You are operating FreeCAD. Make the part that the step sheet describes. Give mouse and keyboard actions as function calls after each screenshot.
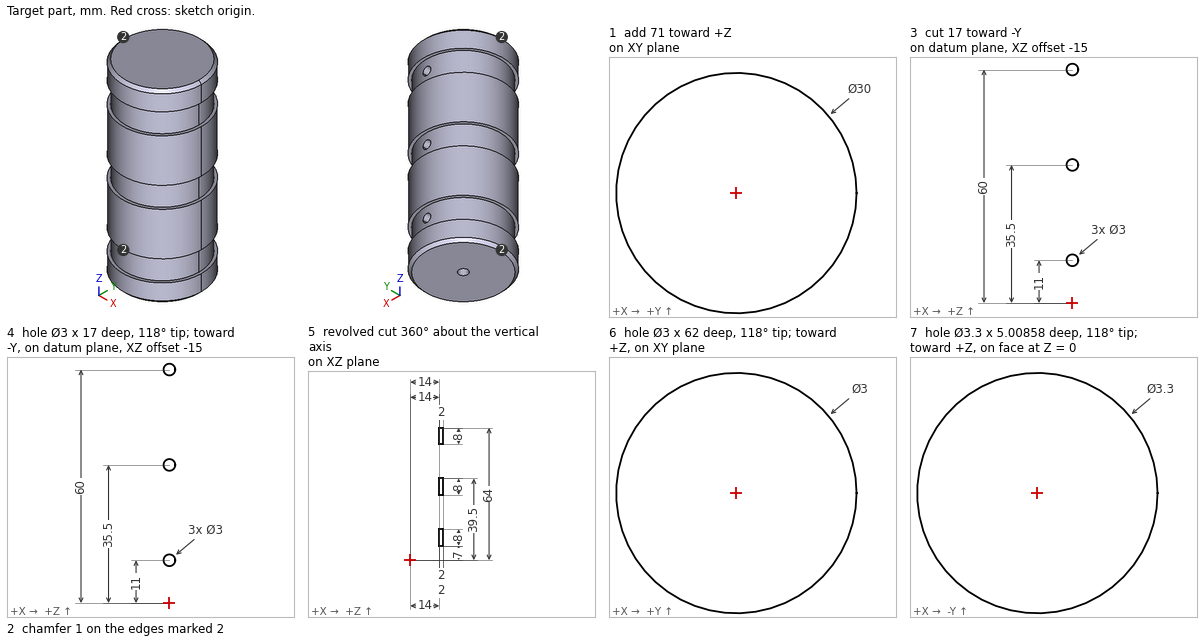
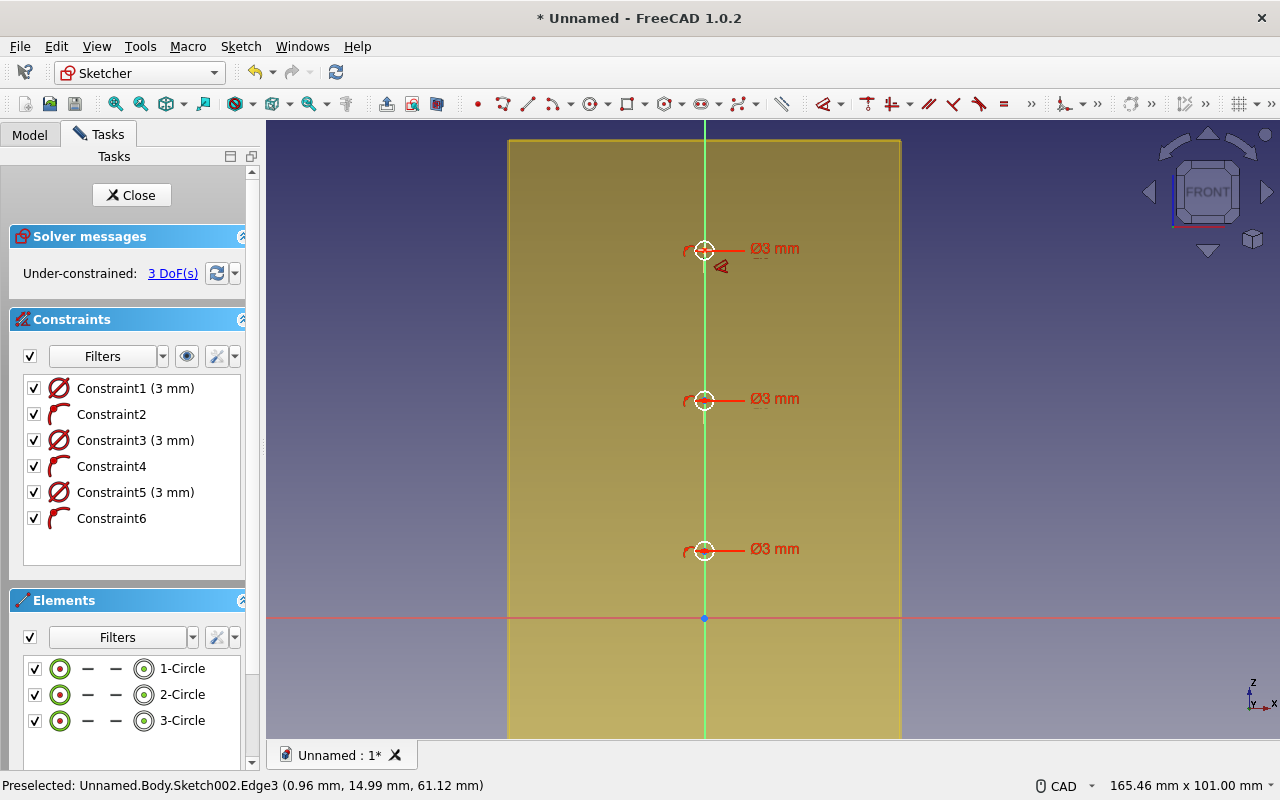
click(705, 551)
click(739, 585)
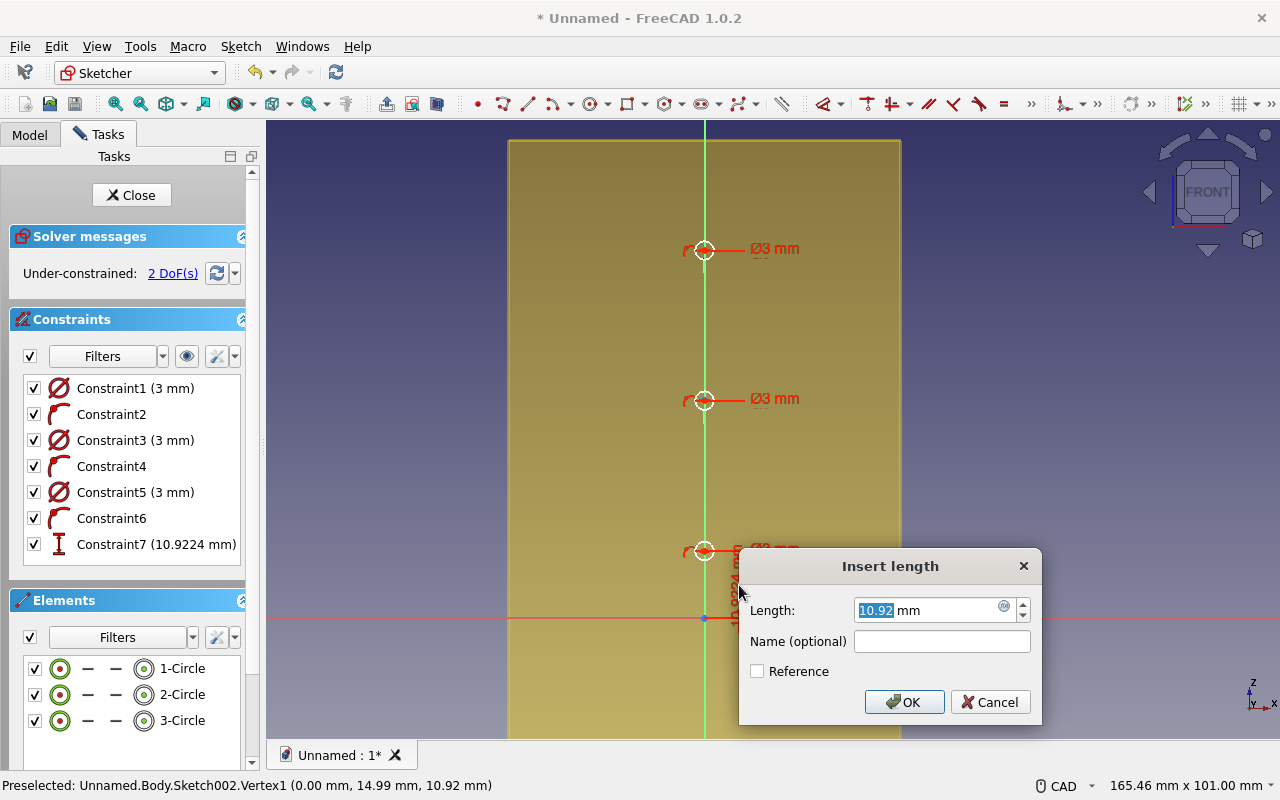
text(11)
key(Return)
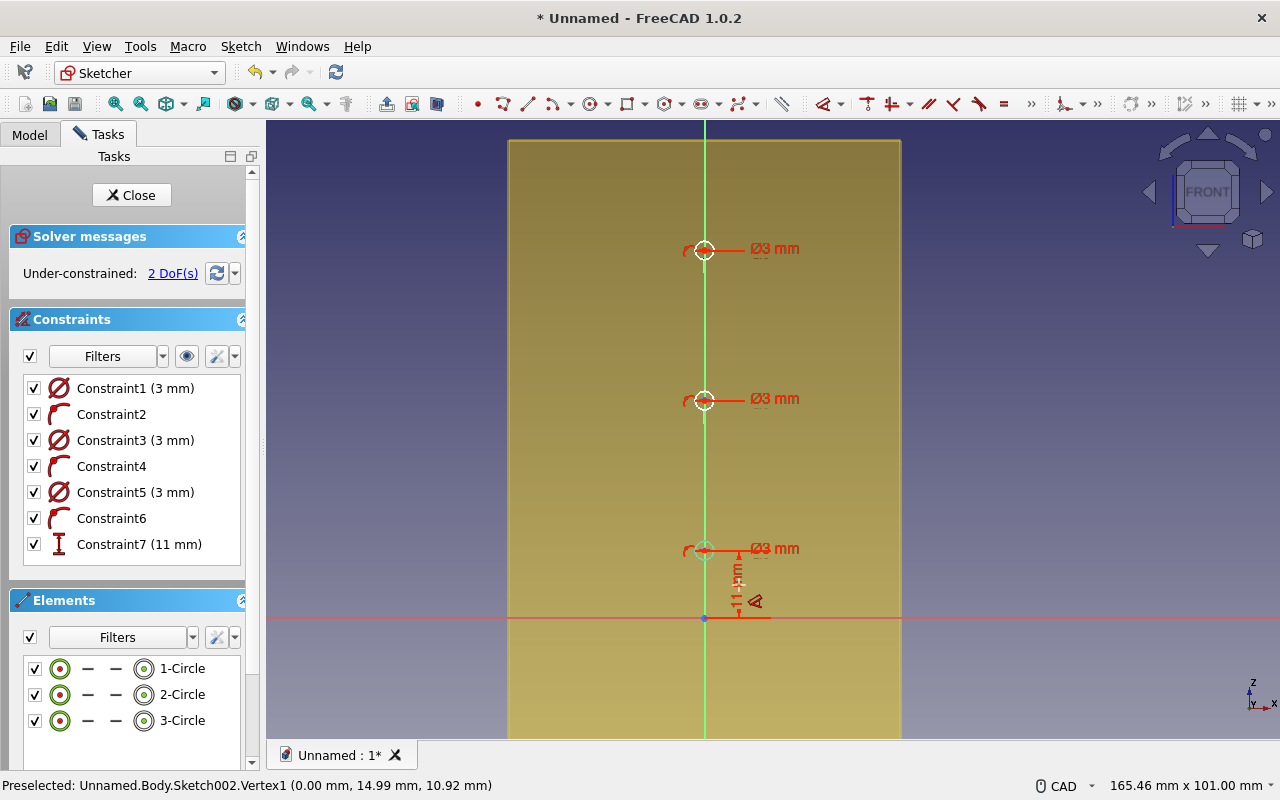
click(705, 251)
click(739, 434)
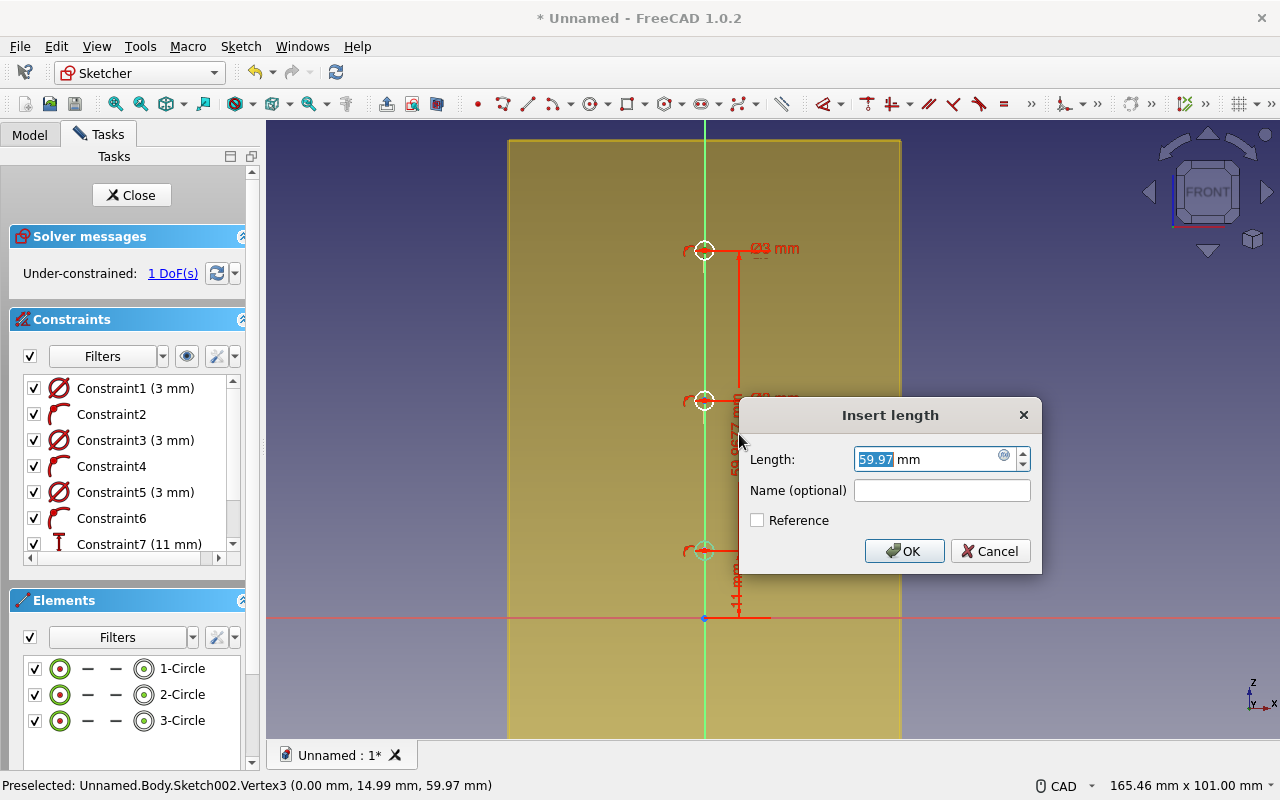
text(60)
key(Return)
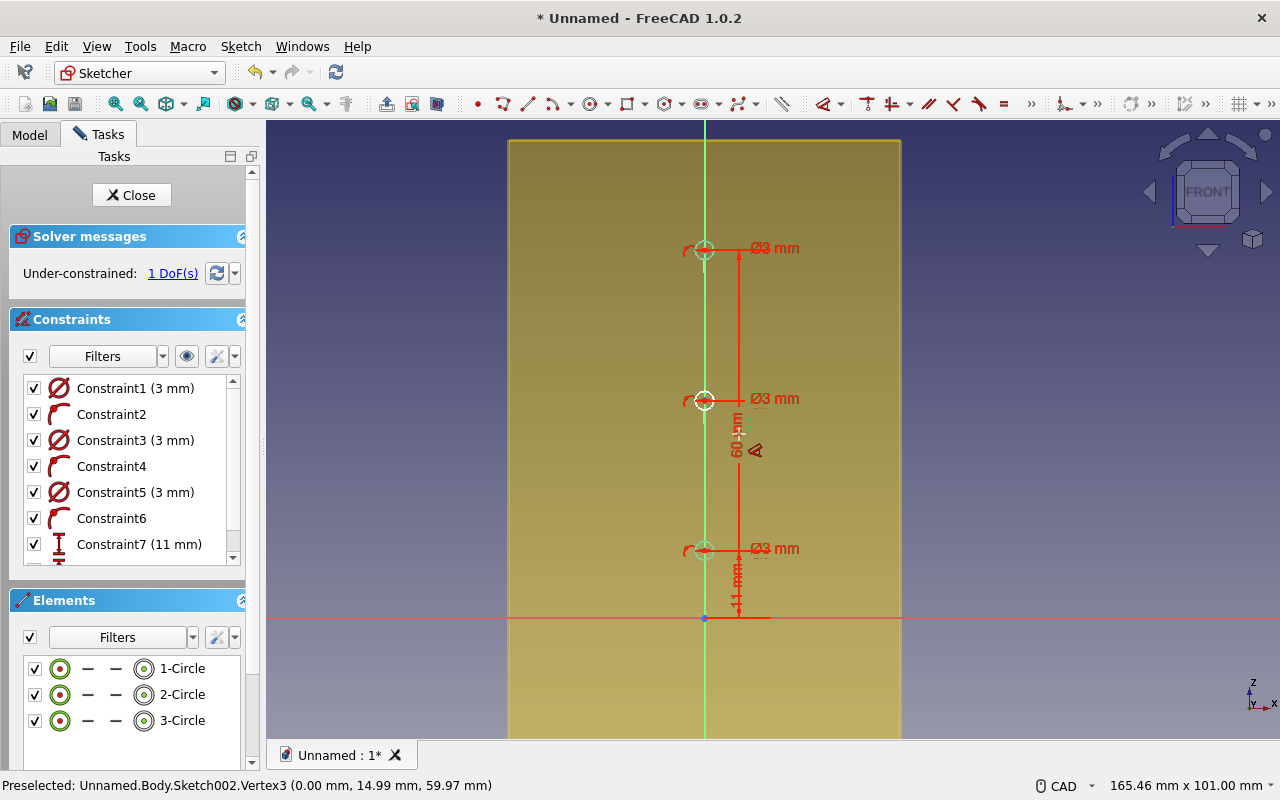
click(705, 401)
click(739, 509)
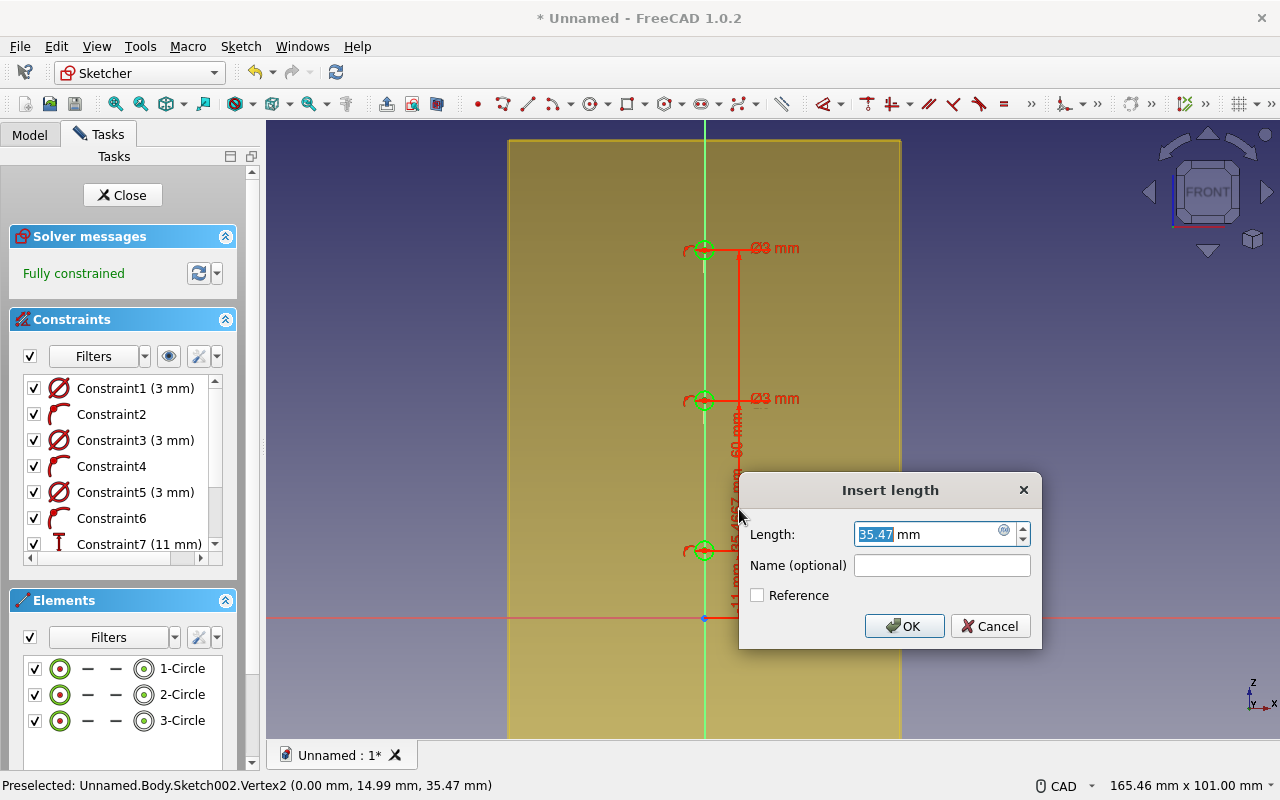
text(35.5)
key(Return)
key(Escape)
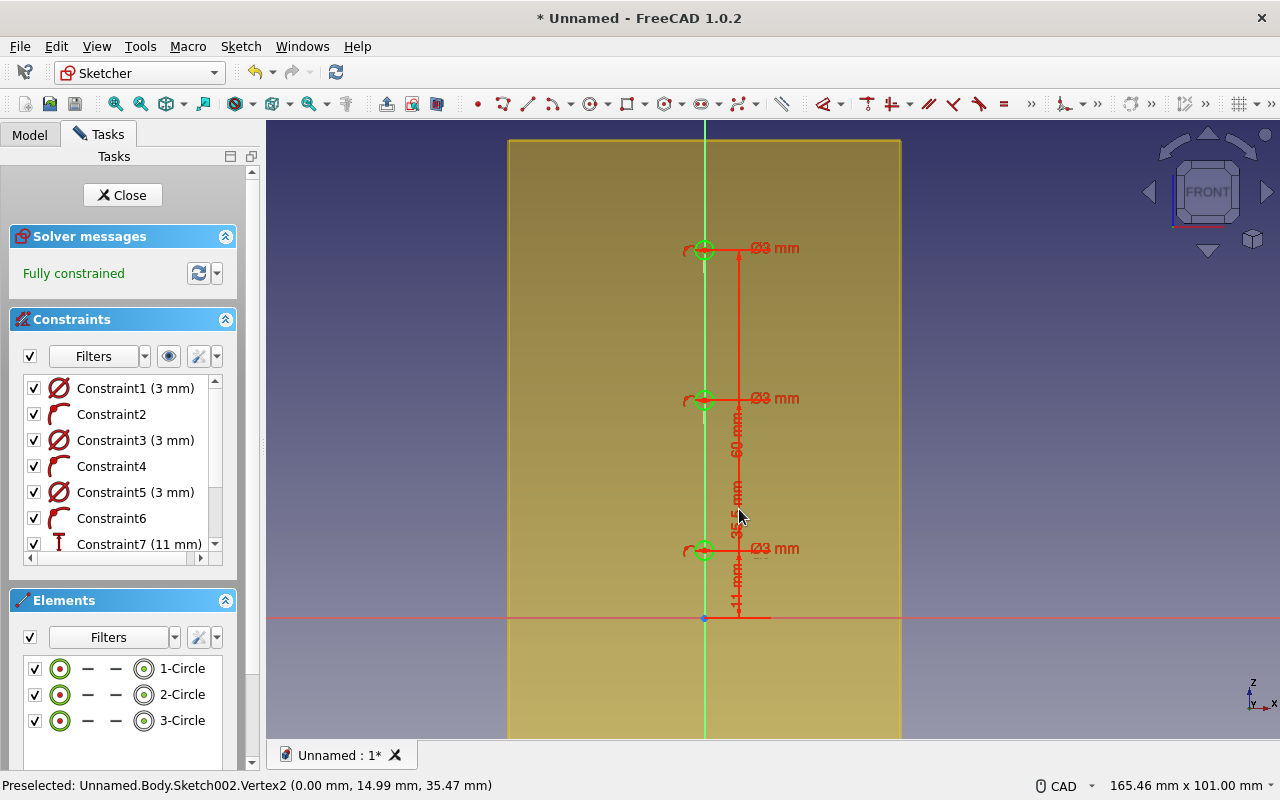
click(123, 195)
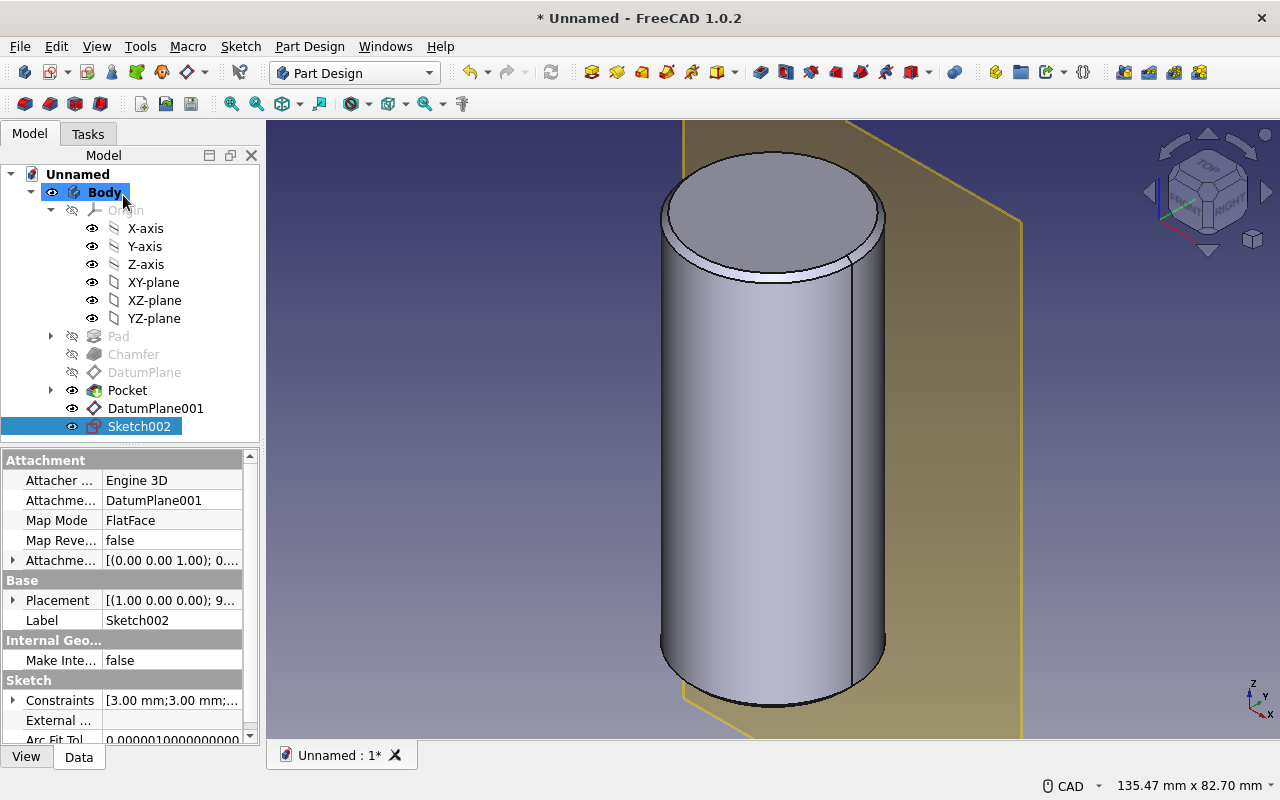
click(786, 72)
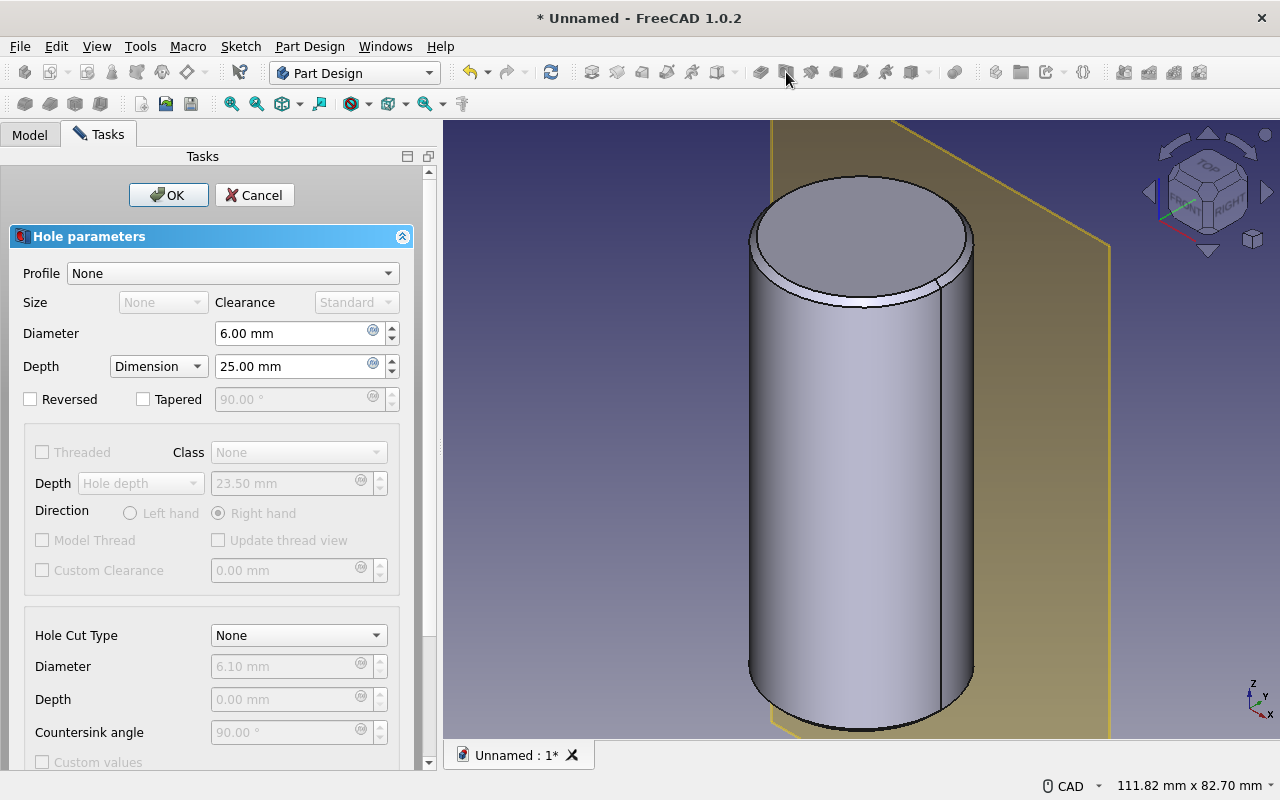
triple_click(300, 334)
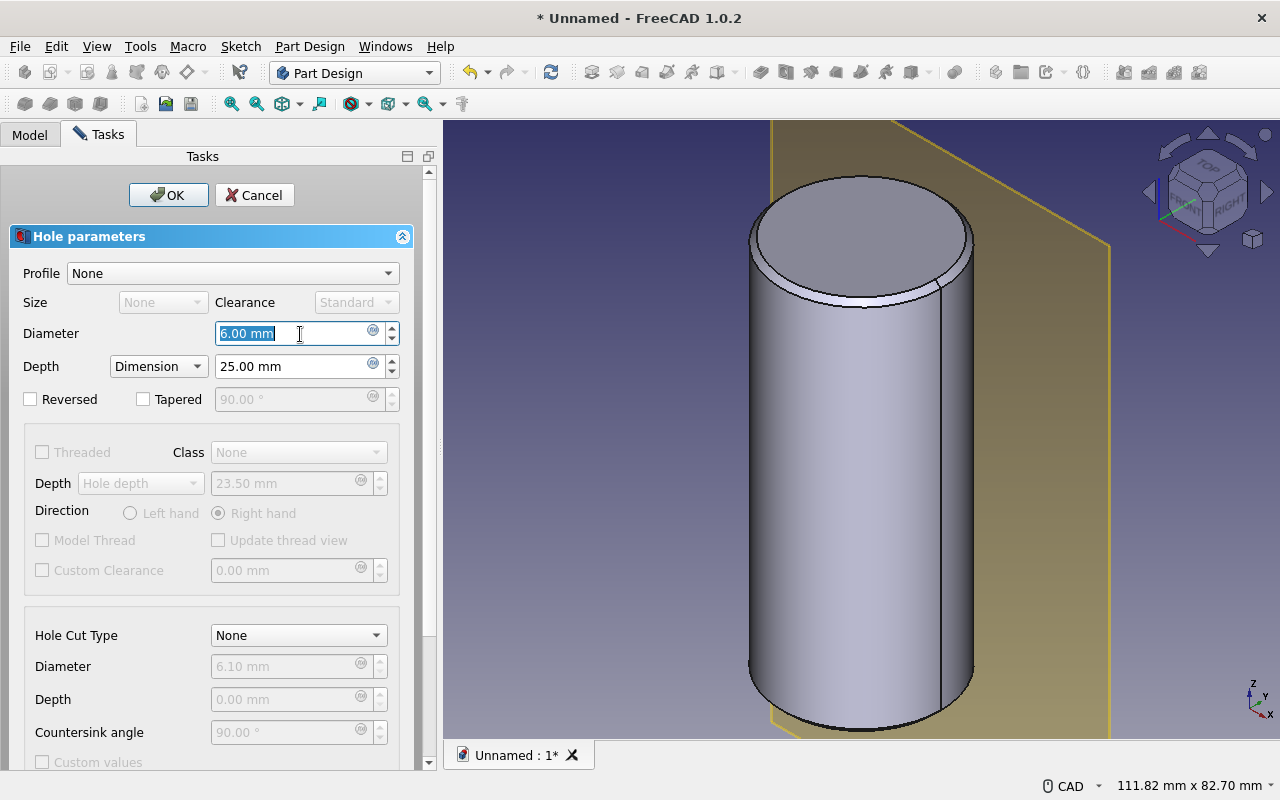
text(3)
key(Tab)